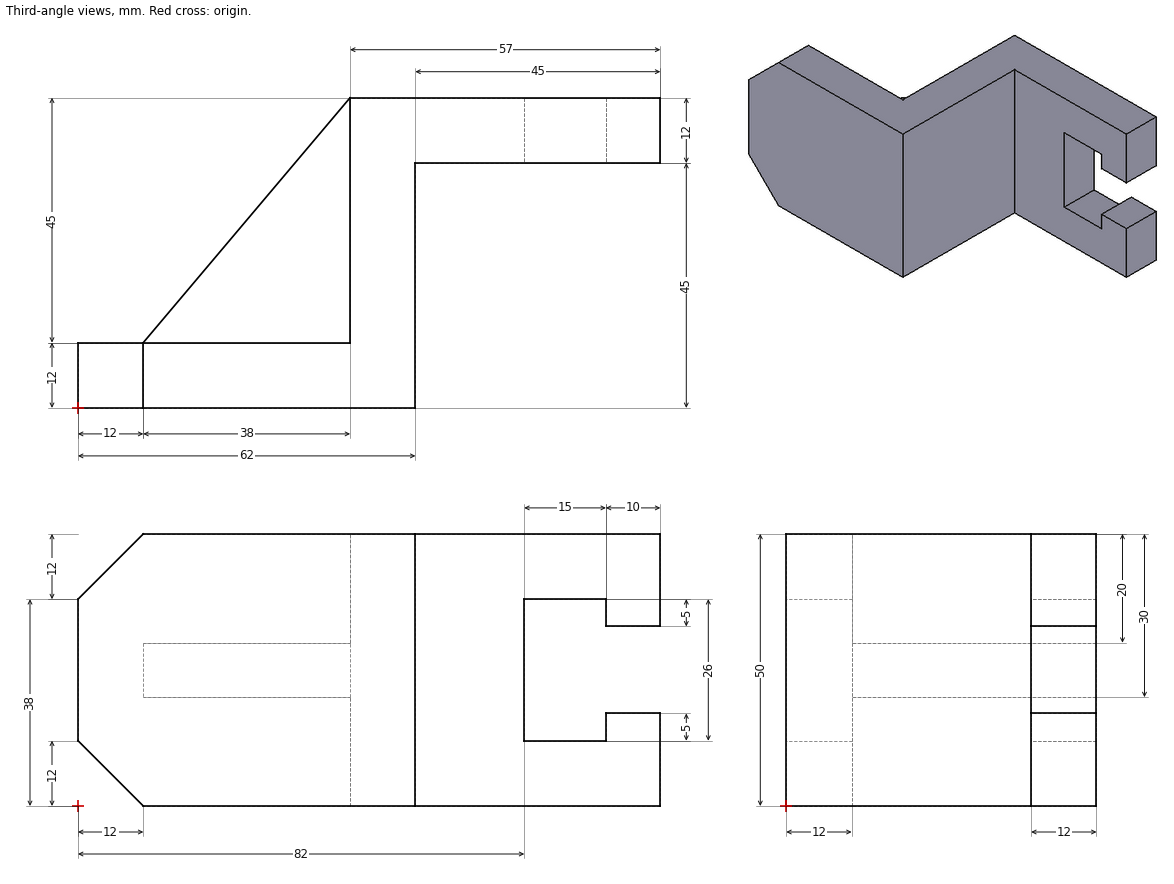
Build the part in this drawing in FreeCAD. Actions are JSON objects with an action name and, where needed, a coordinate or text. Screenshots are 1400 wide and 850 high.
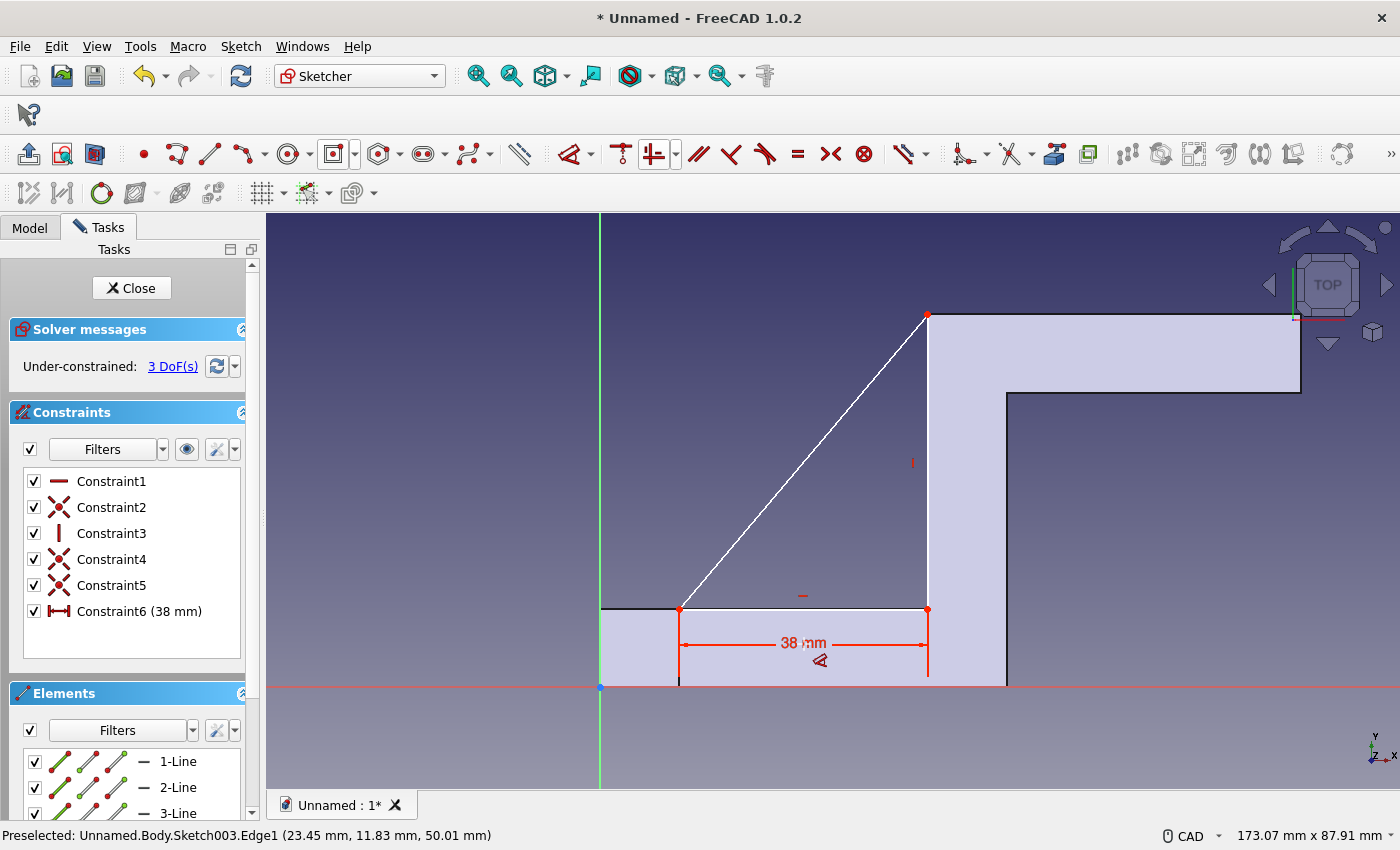
{"action": "left_click", "coordinate": [928, 521]}
{"action": "left_click", "coordinate": [962, 462]}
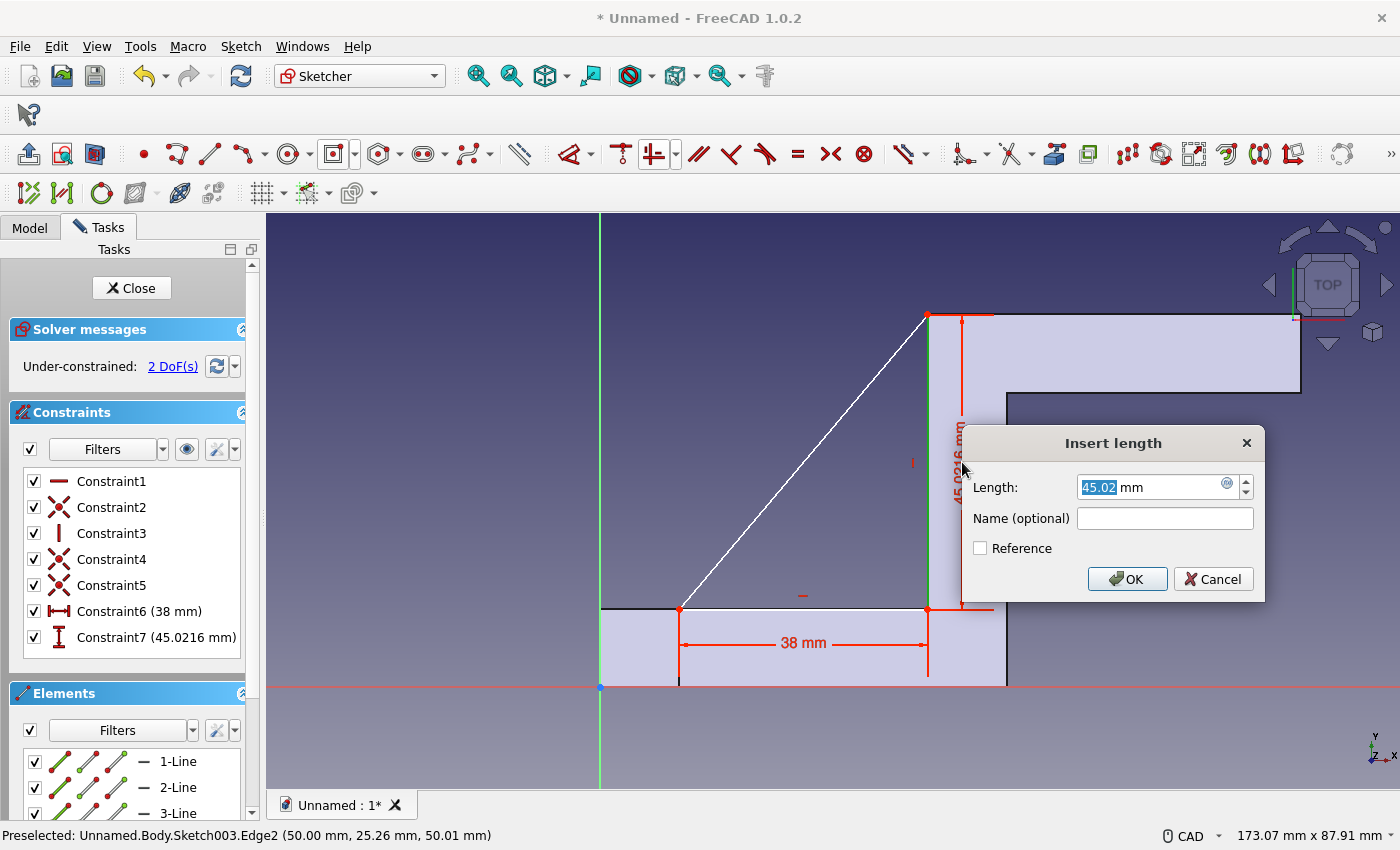
{"action": "type", "text": "45"}
{"action": "key", "text": "Return"}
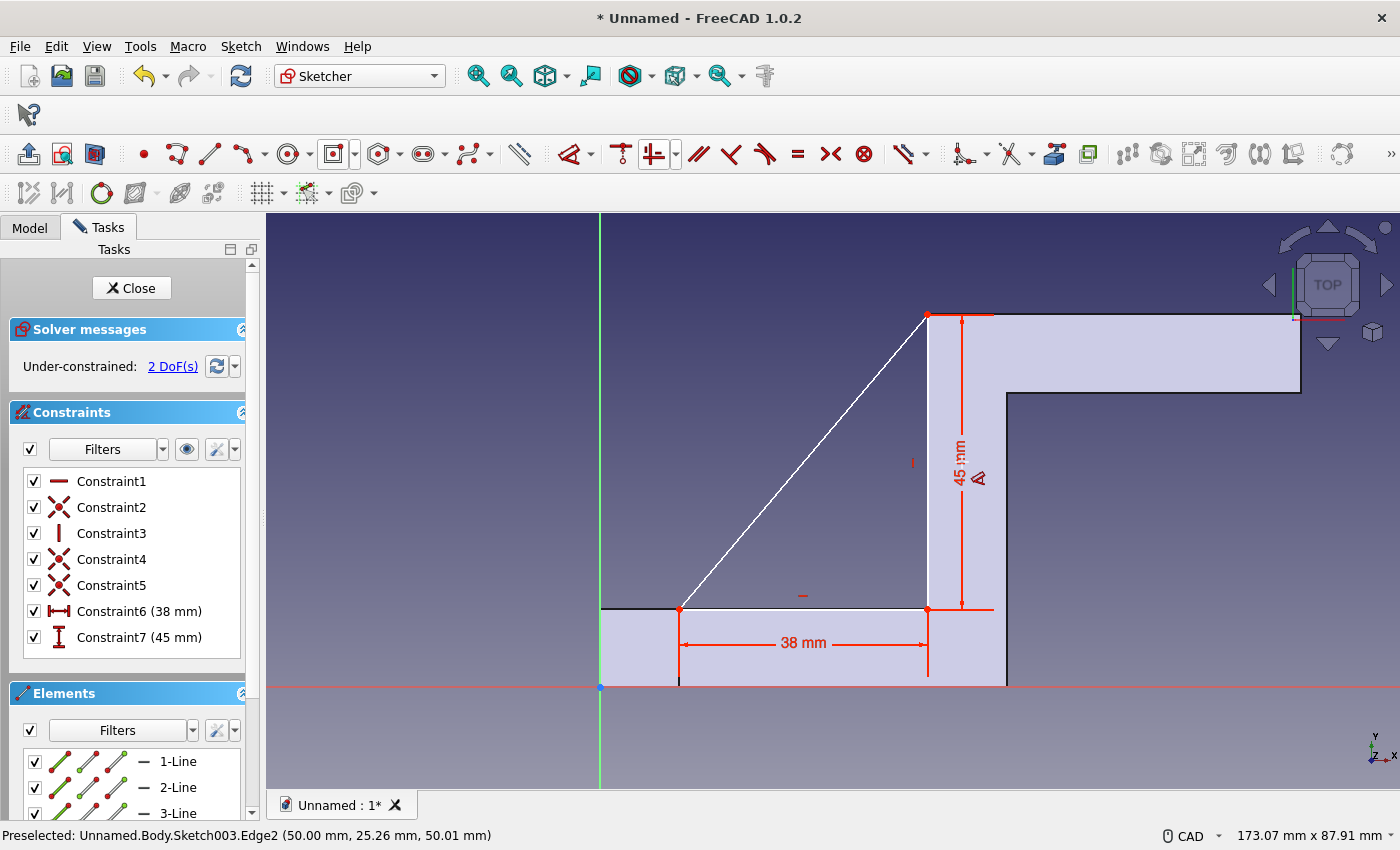
{"action": "left_click", "coordinate": [679, 610]}
{"action": "left_click", "coordinate": [640, 721]}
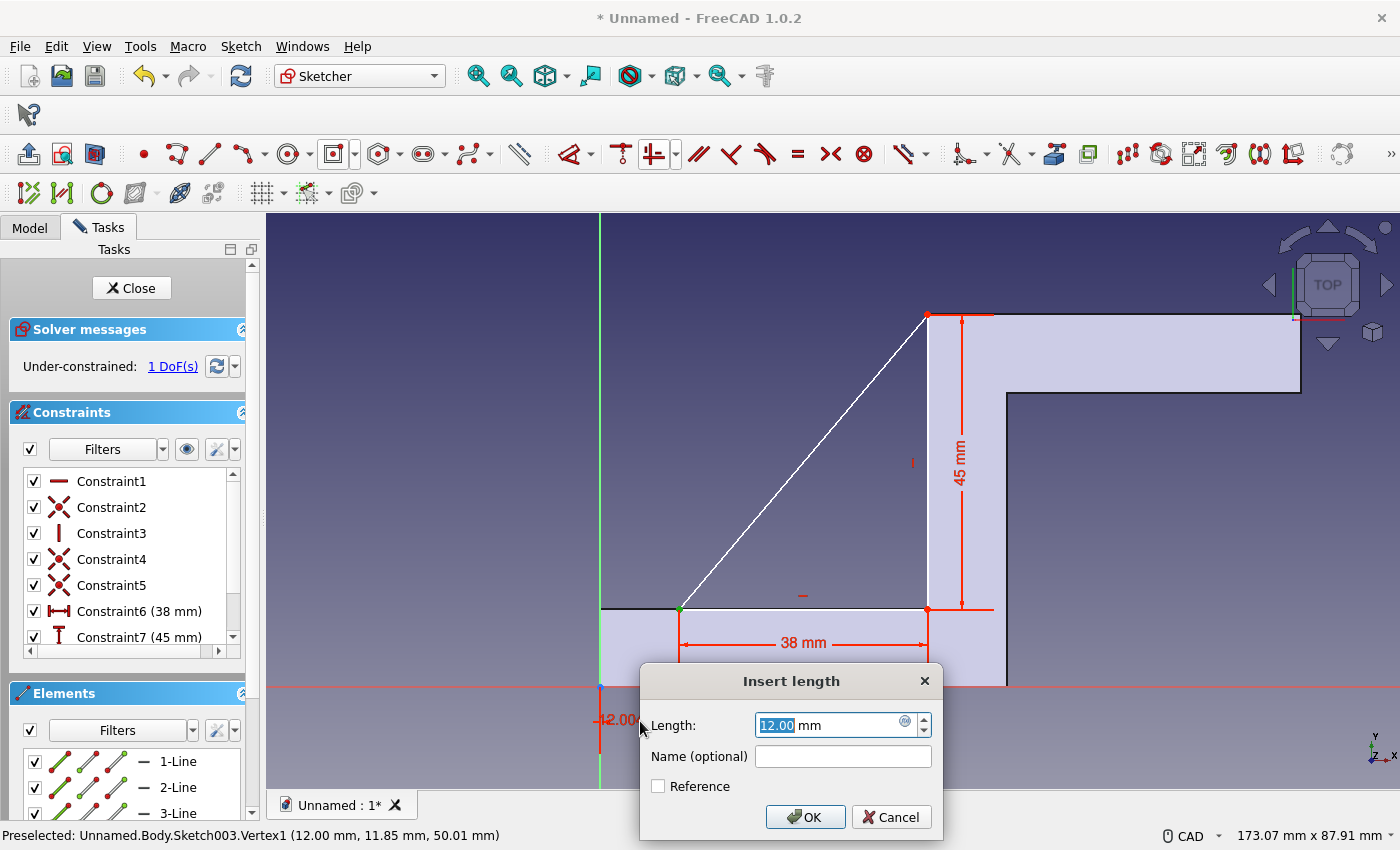
{"action": "type", "text": "12"}
{"action": "key", "text": "Return"}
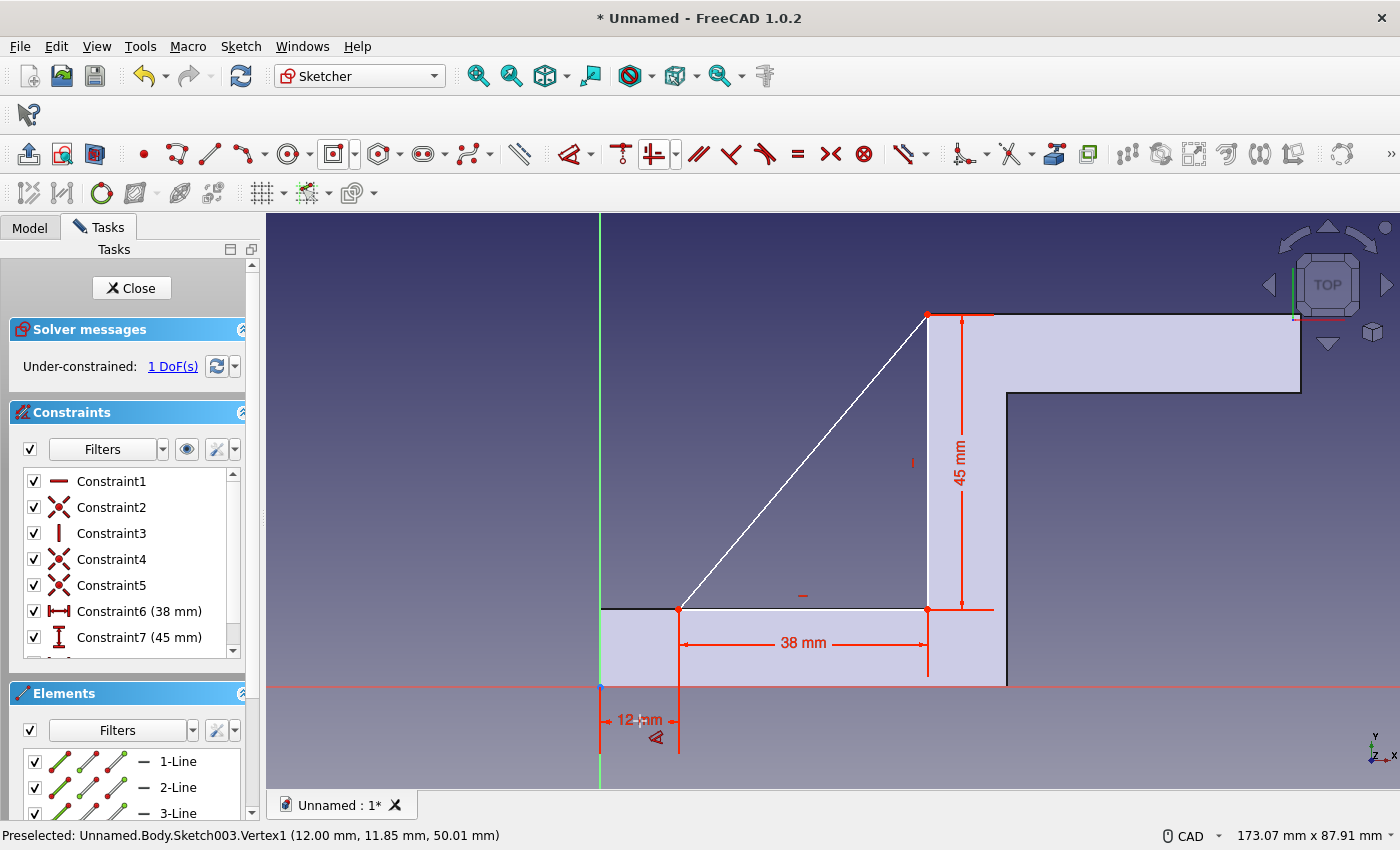
{"action": "left_click", "coordinate": [679, 610]}
{"action": "left_click", "coordinate": [566, 649]}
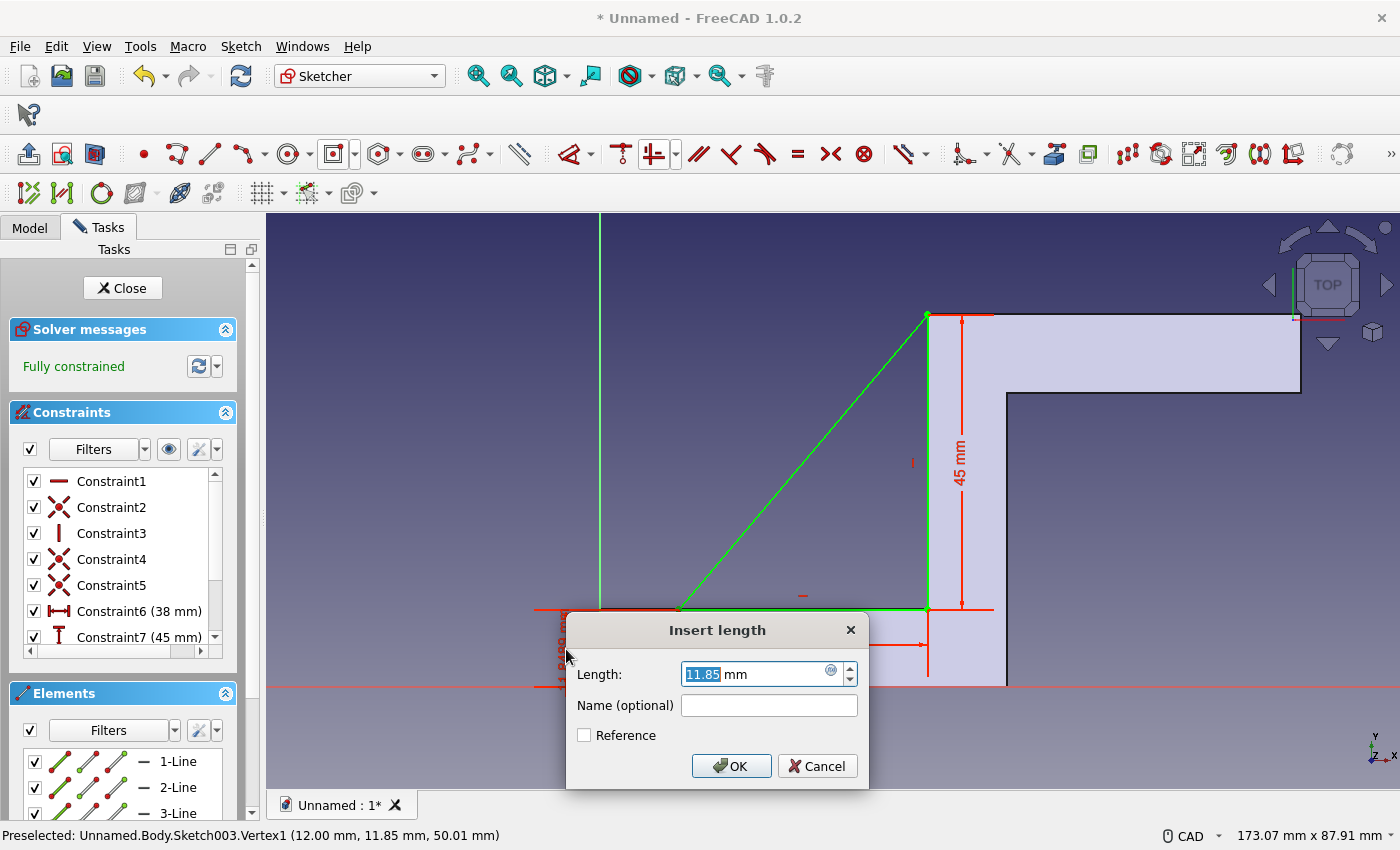
{"action": "type", "text": "12"}
{"action": "key", "text": "Return"}
{"action": "key", "text": "Escape"}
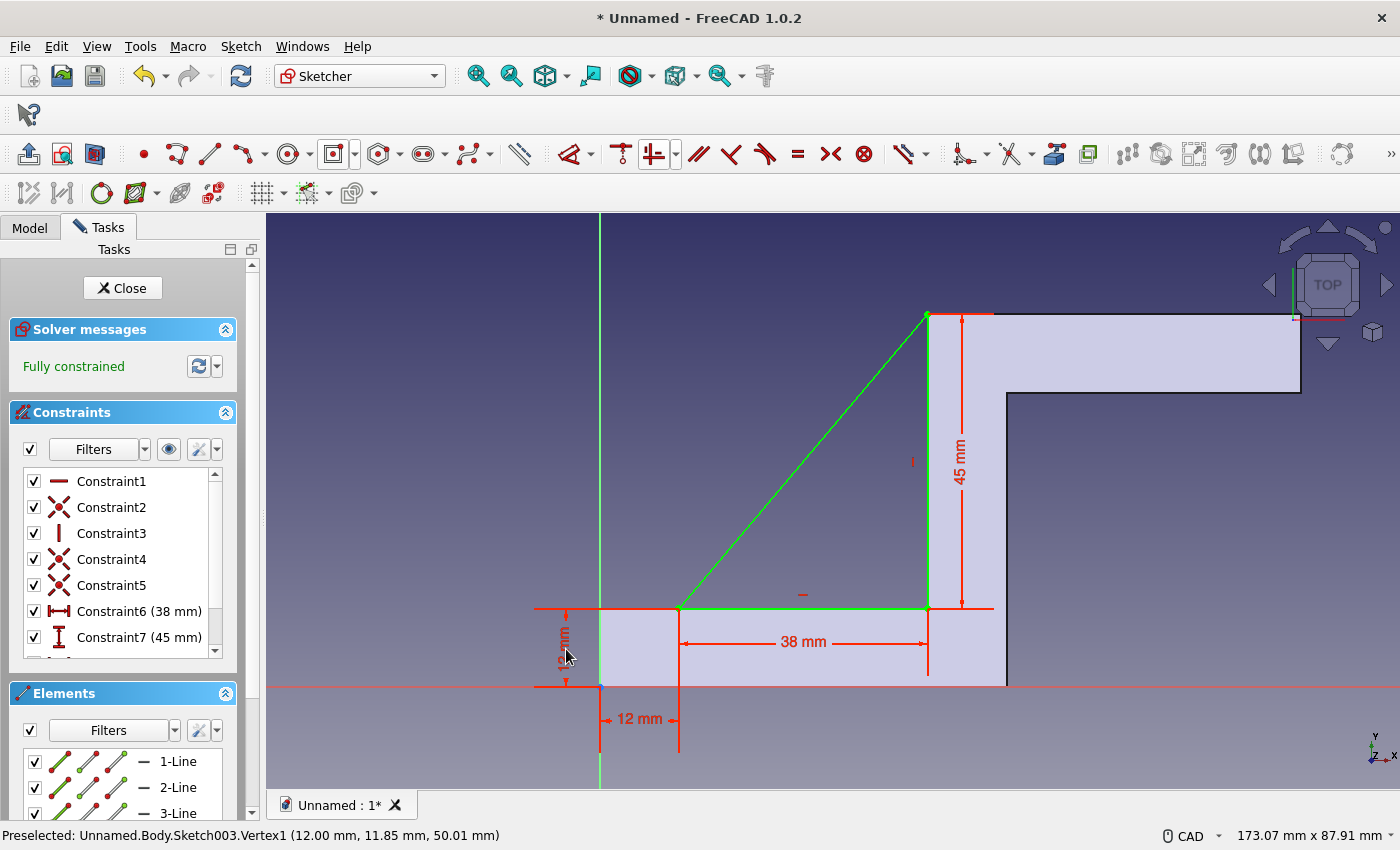
{"action": "left_click", "coordinate": [123, 288]}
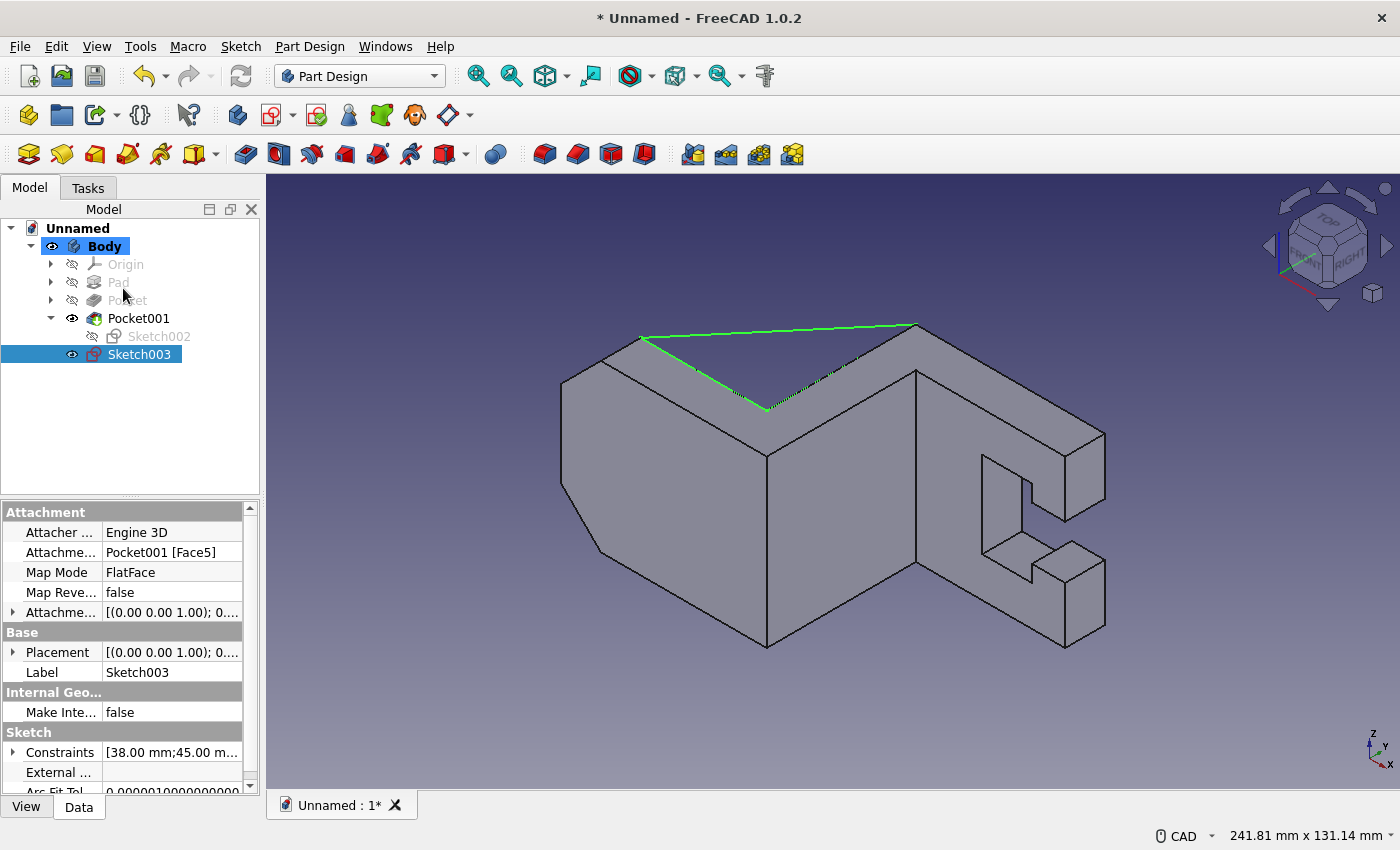
{"action": "left_click", "coordinate": [29, 154]}